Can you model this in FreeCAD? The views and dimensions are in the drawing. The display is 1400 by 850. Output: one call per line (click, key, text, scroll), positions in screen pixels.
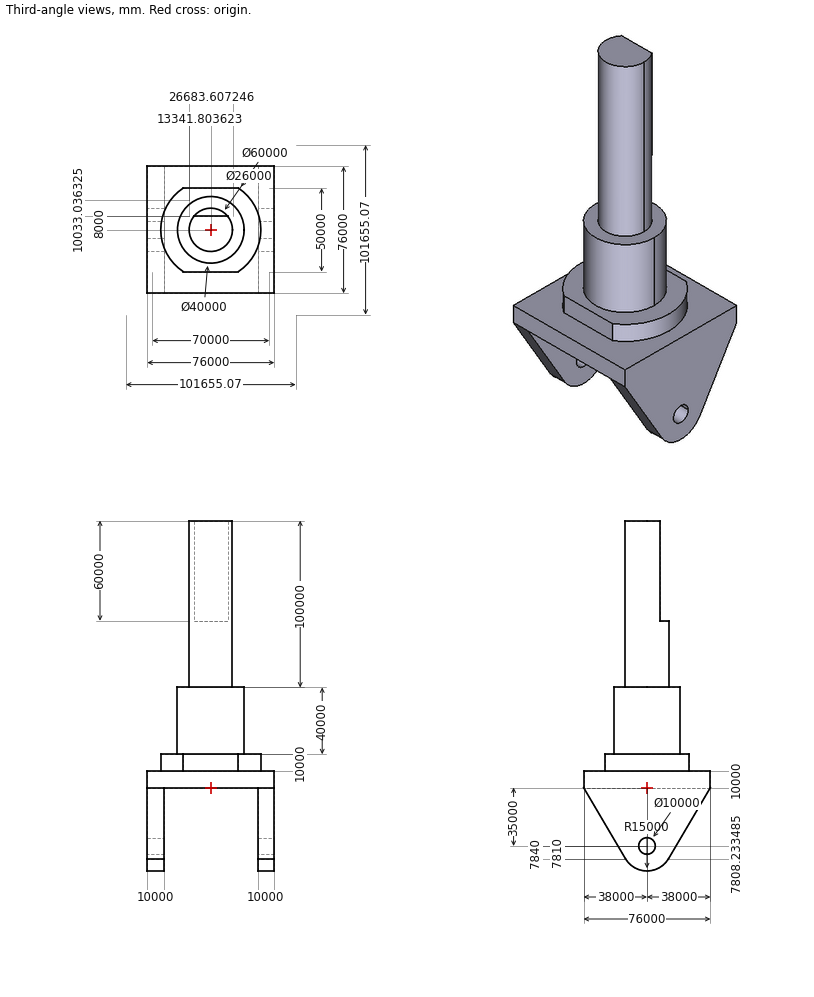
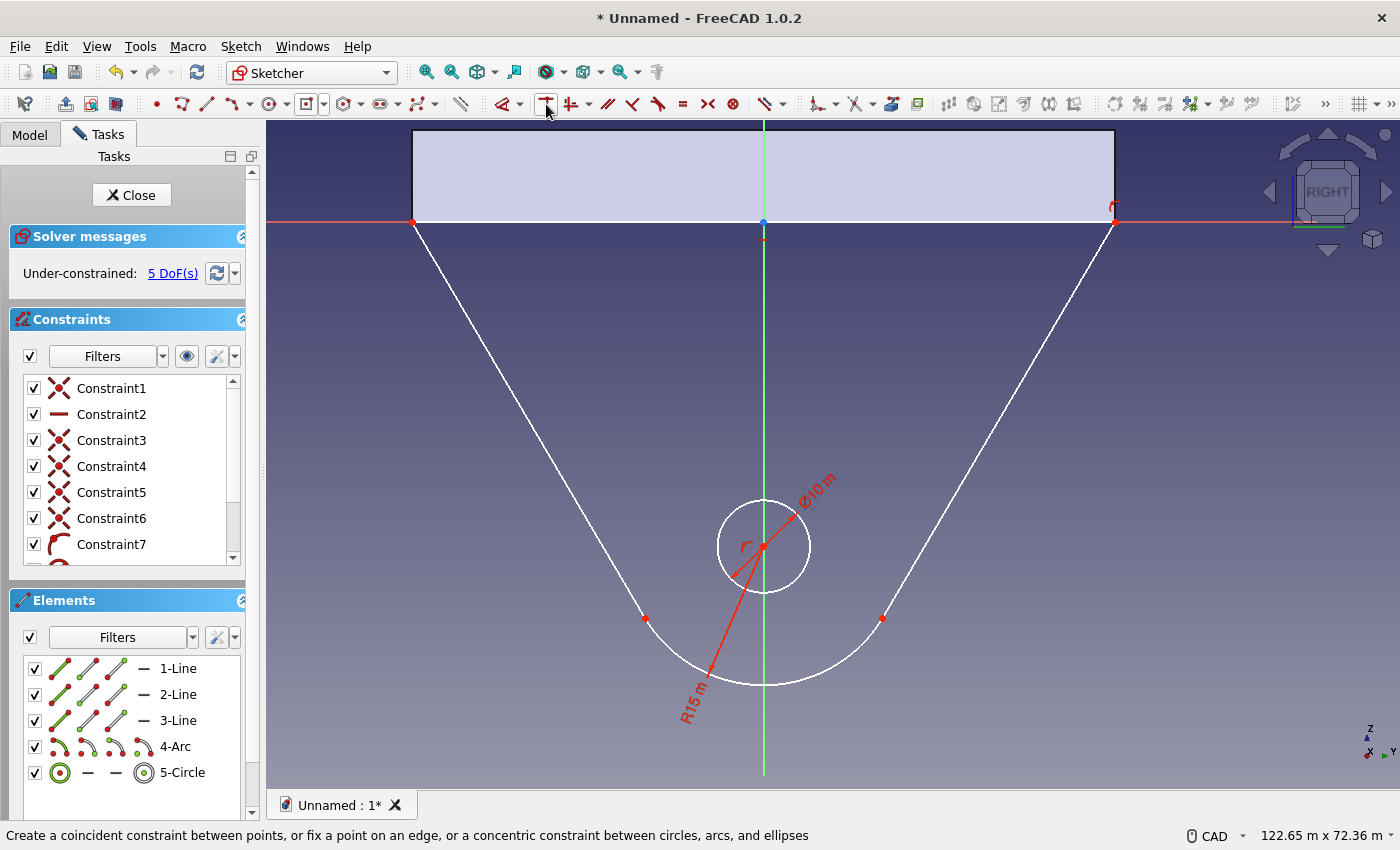
click(502, 104)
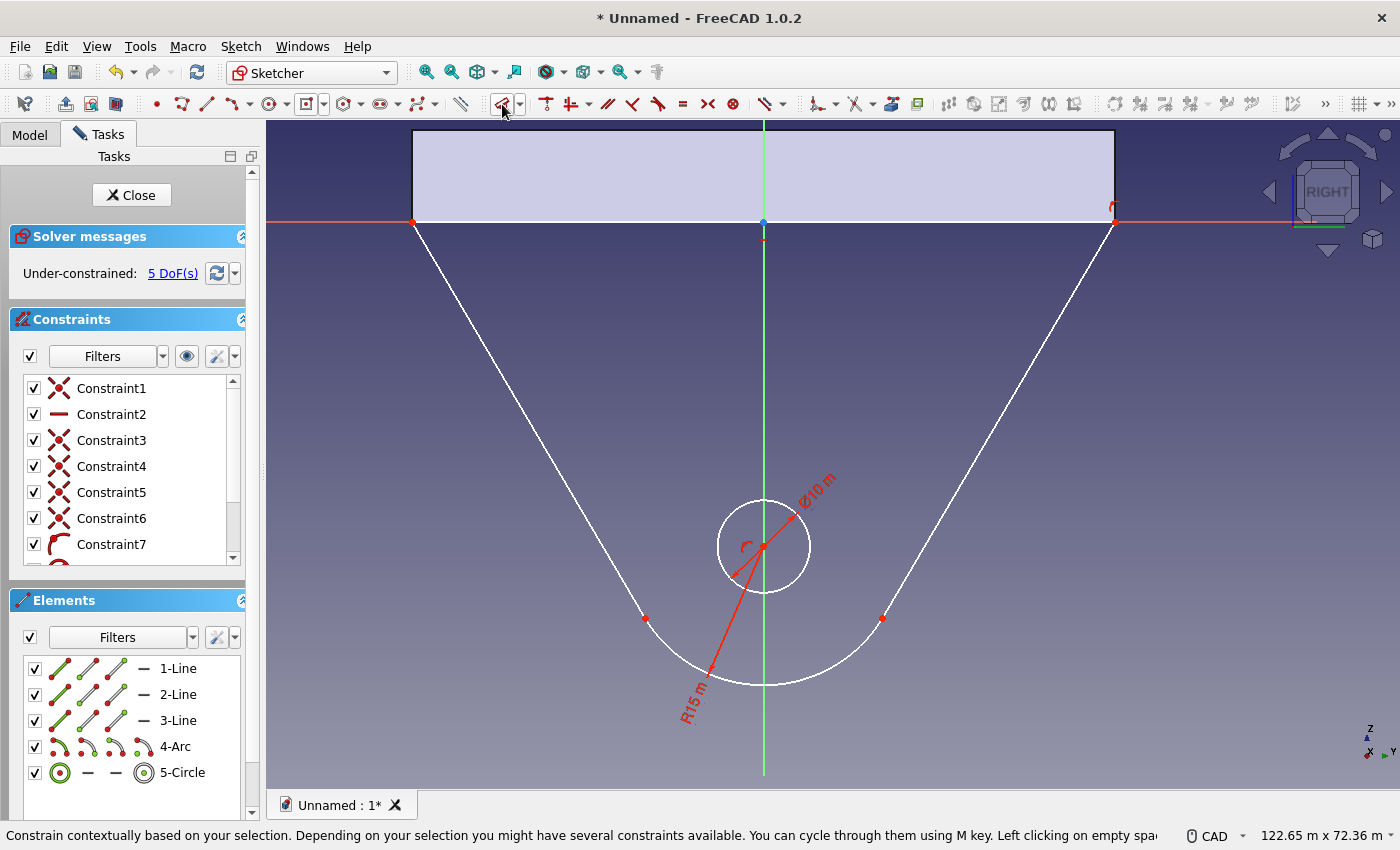
click(904, 222)
click(602, 188)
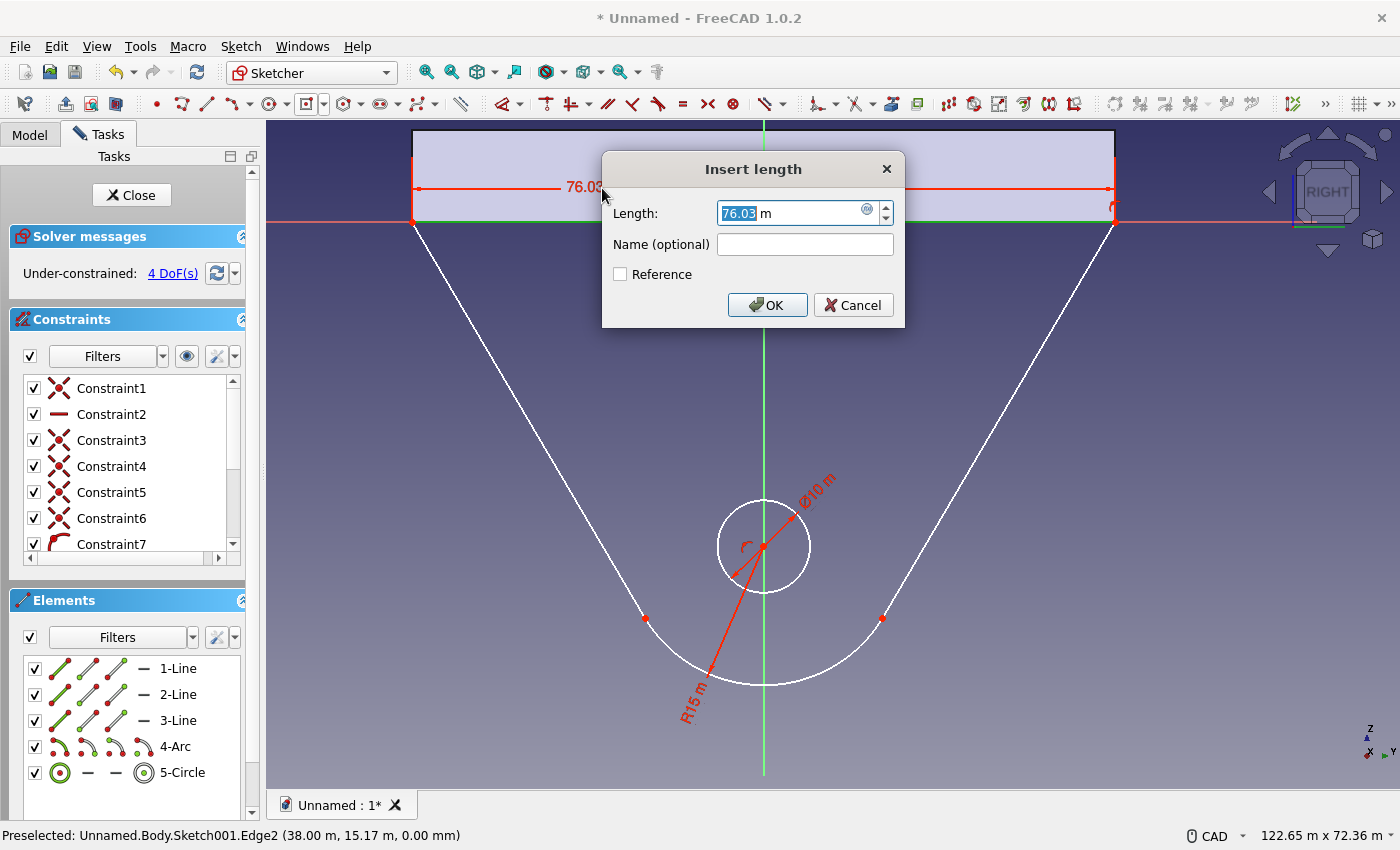
key(ctrl+a)
text(76000 mm)
key(Return)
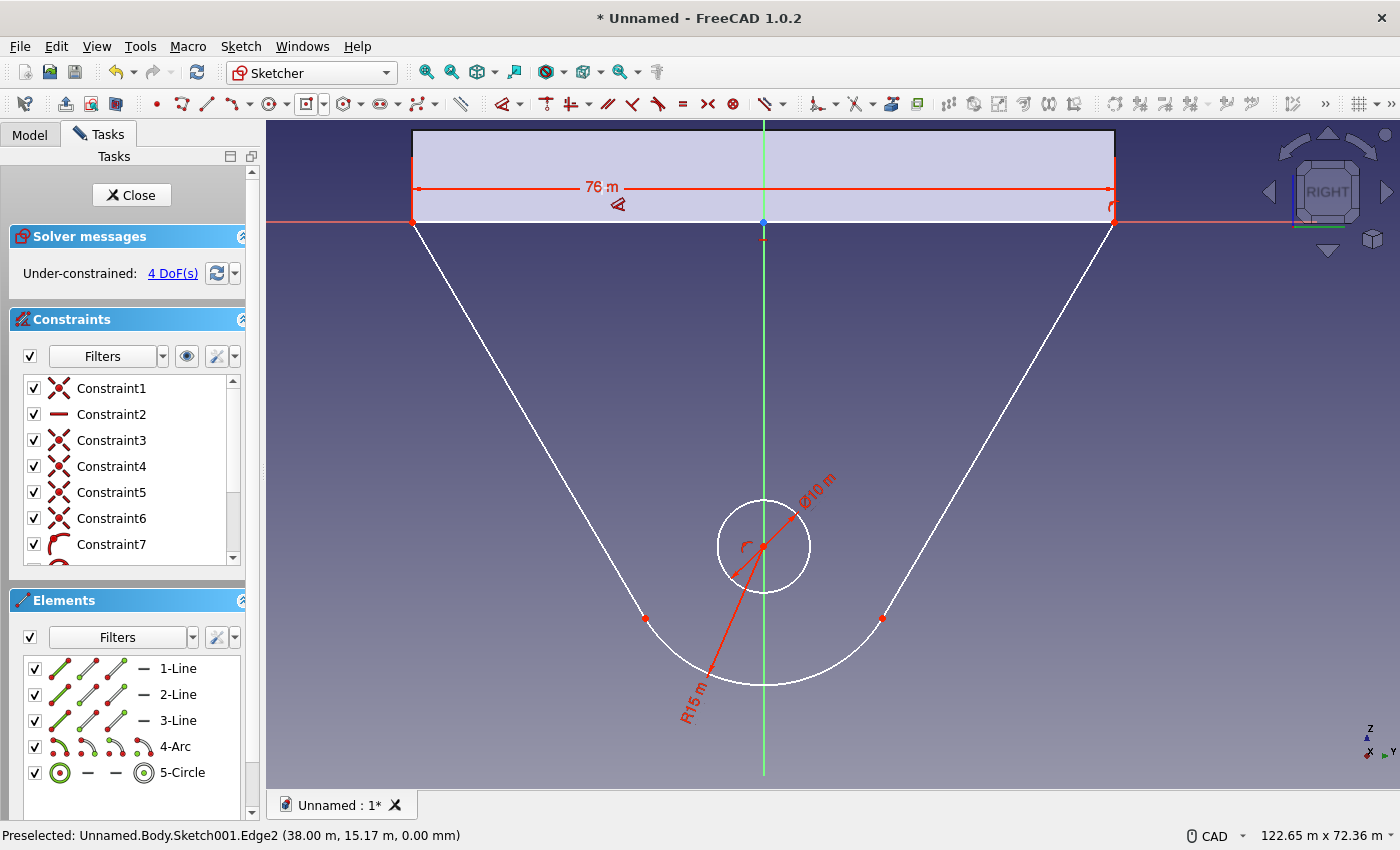
click(764, 547)
click(798, 385)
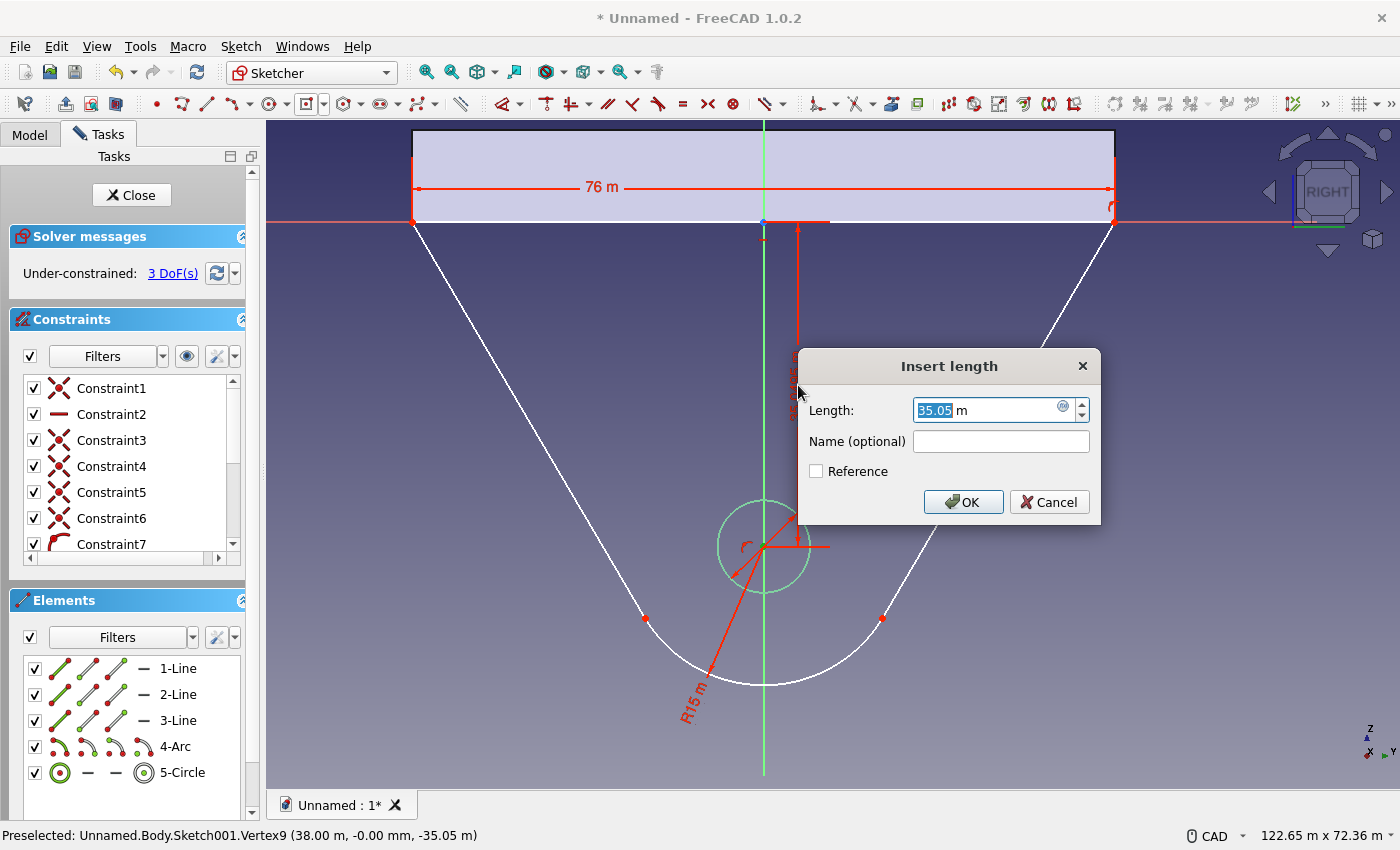
key(ctrl+a)
text(35000 mm)
key(Return)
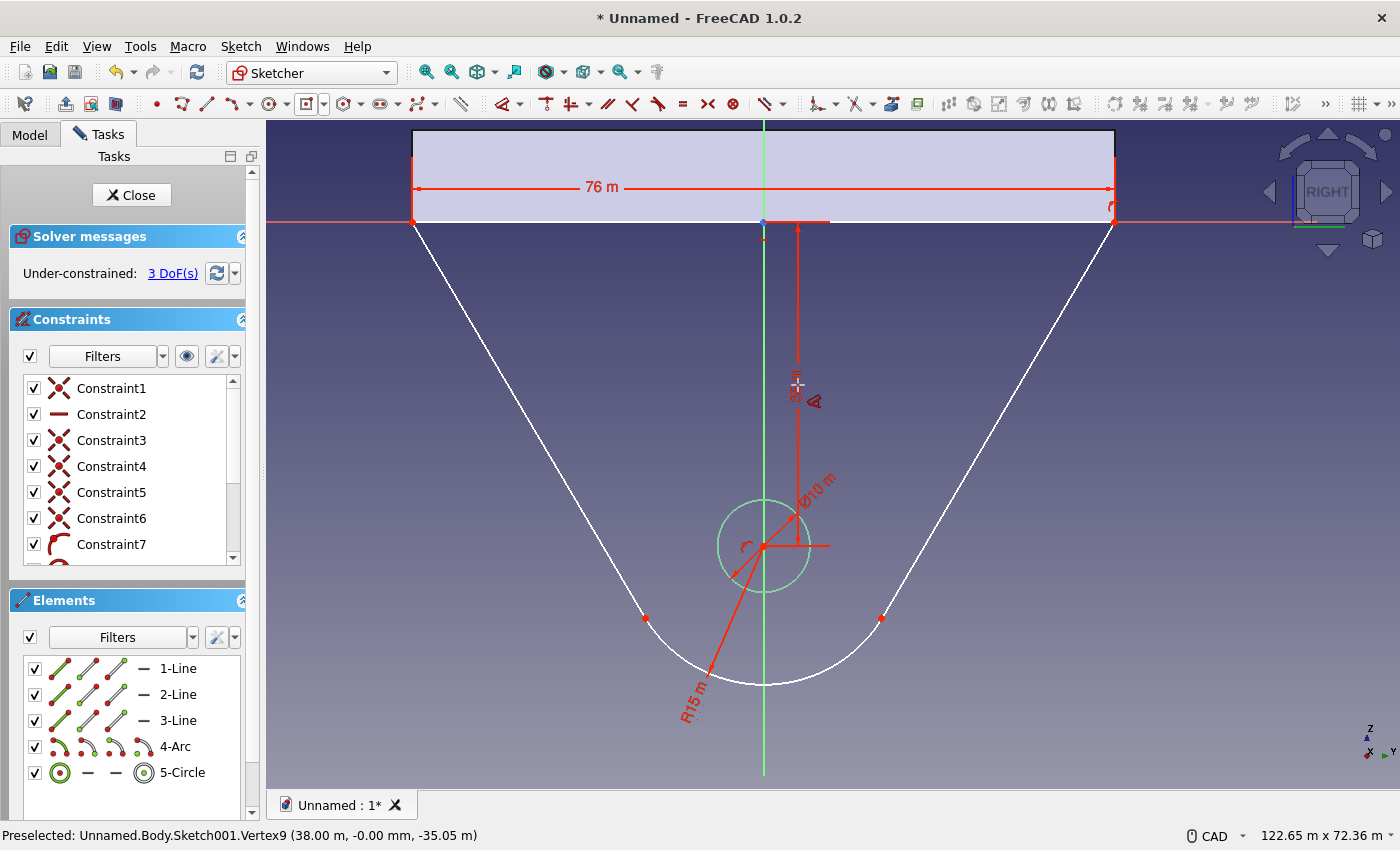
click(646, 619)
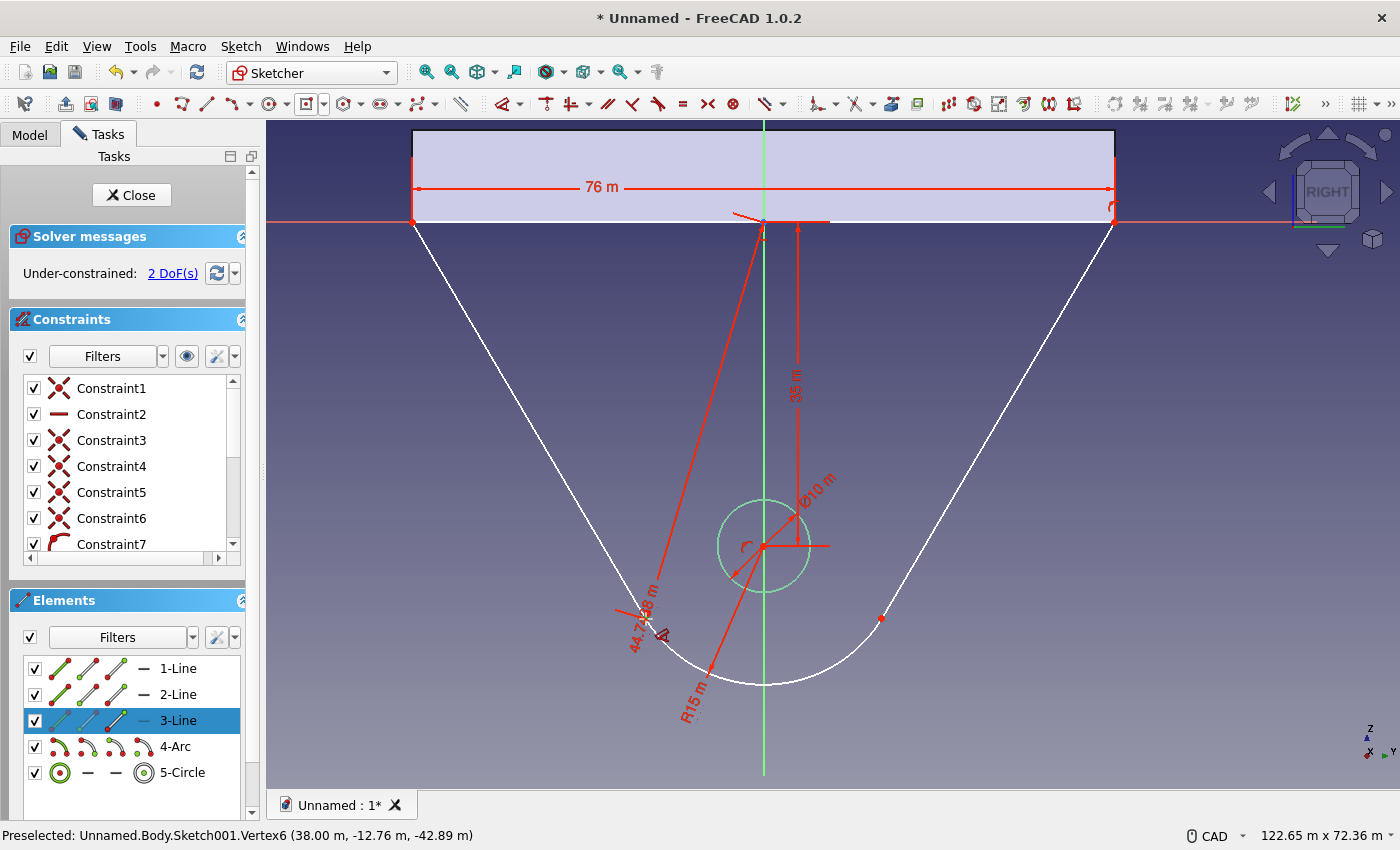
click(764, 546)
click(612, 599)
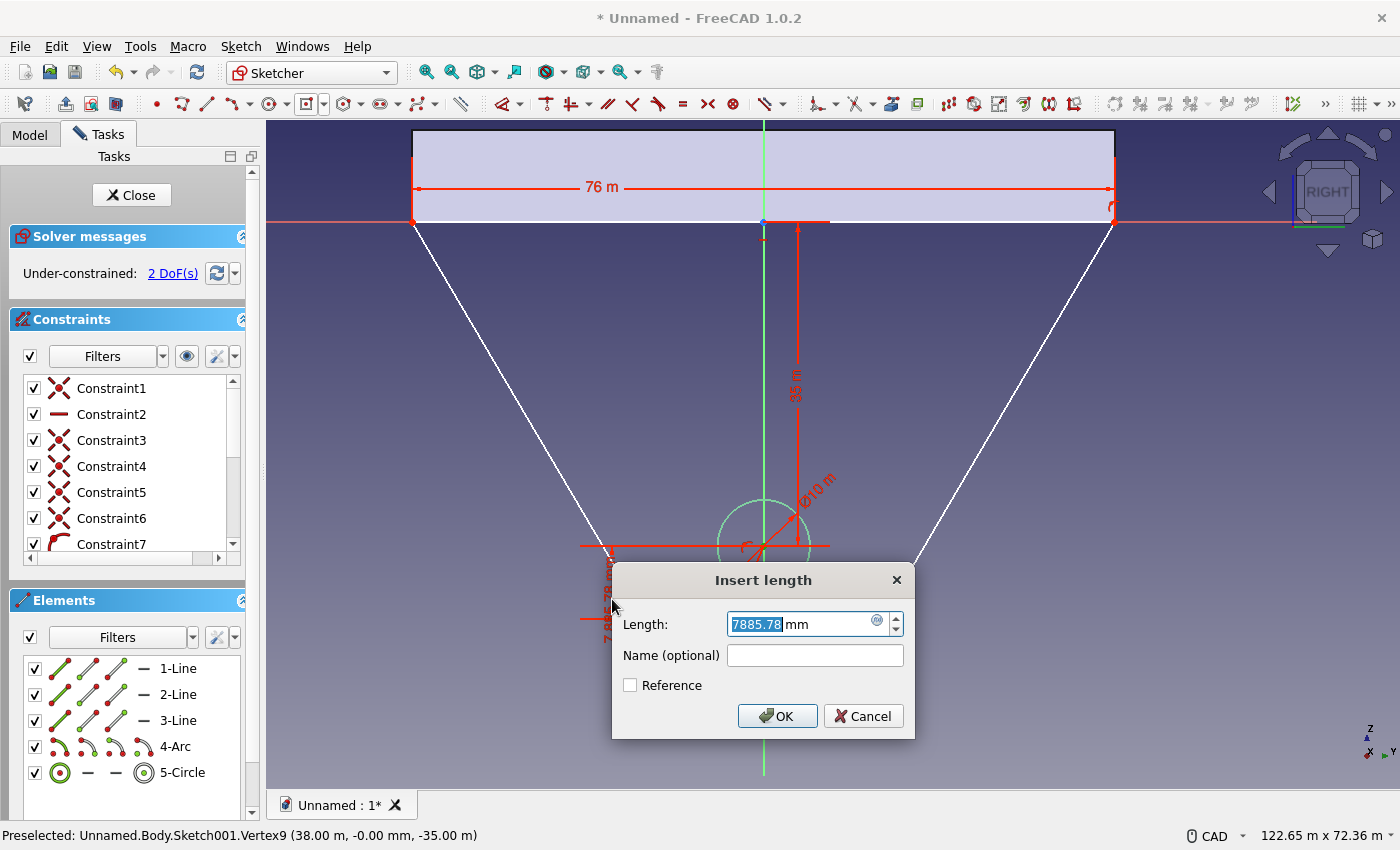
text(7810)
key(Return)